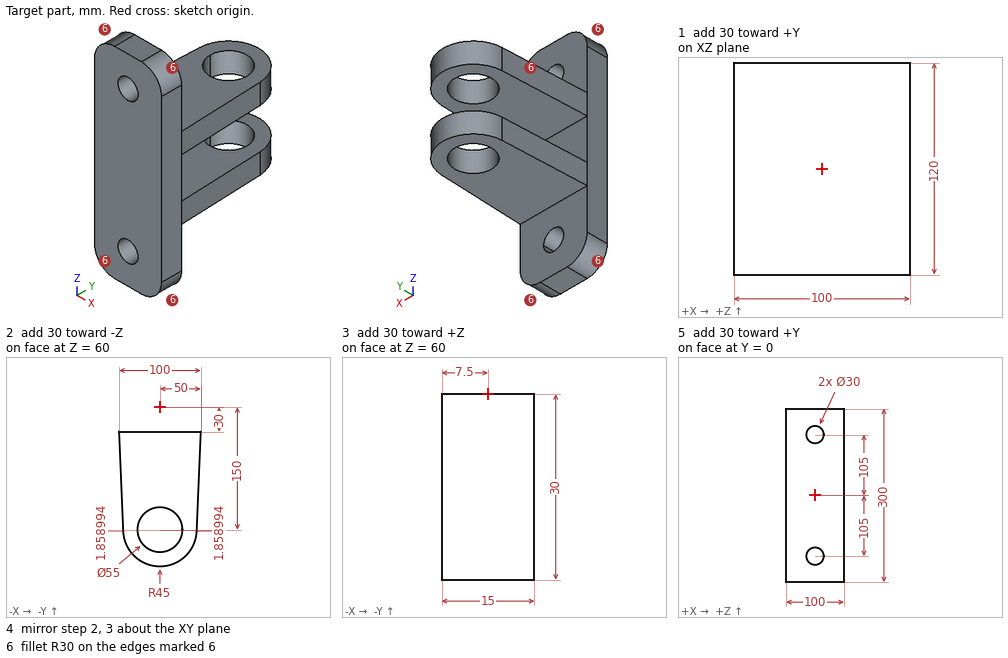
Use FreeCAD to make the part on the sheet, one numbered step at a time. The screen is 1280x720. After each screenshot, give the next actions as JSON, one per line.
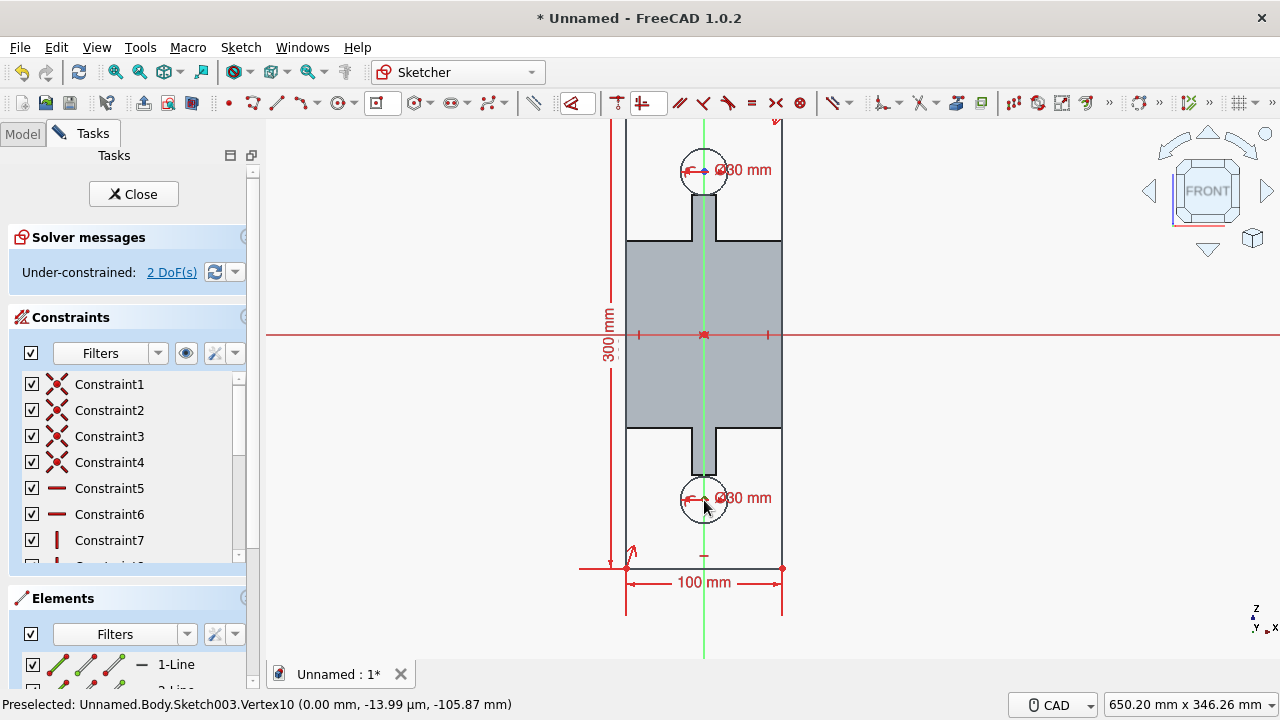
{"action": "left_click", "coordinate": [590, 104]}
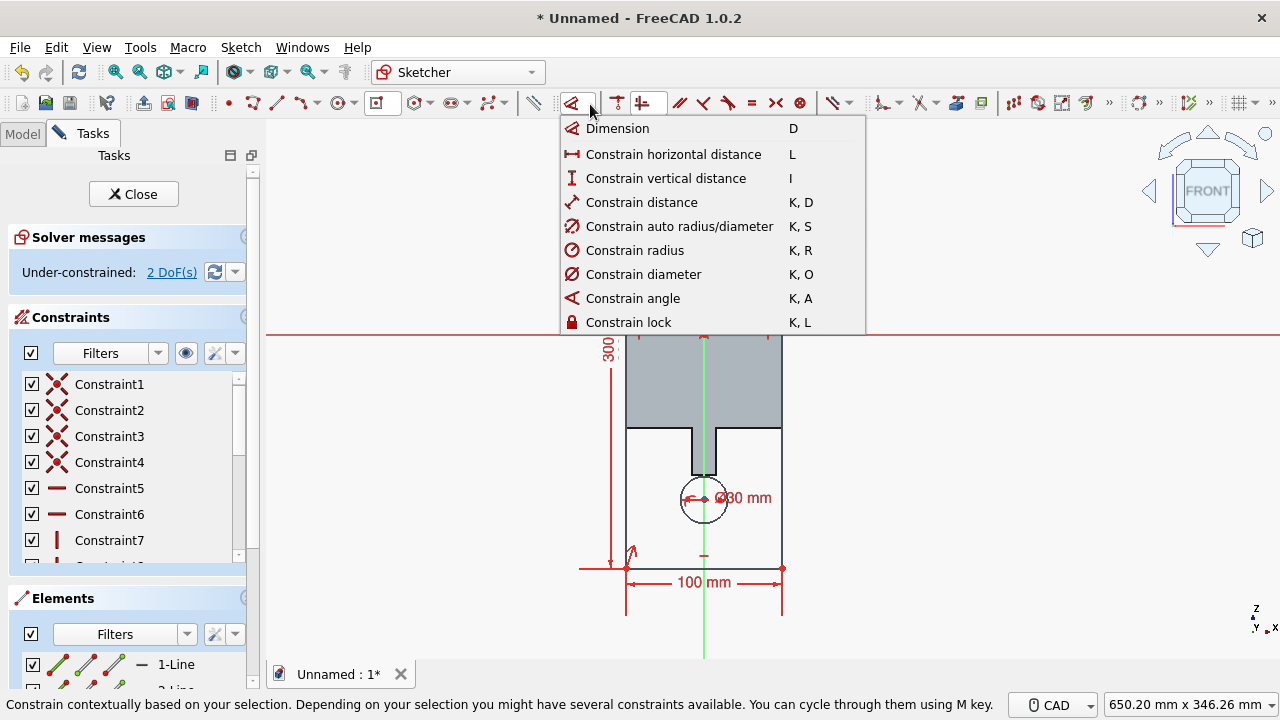
{"action": "left_click", "coordinate": [713, 178]}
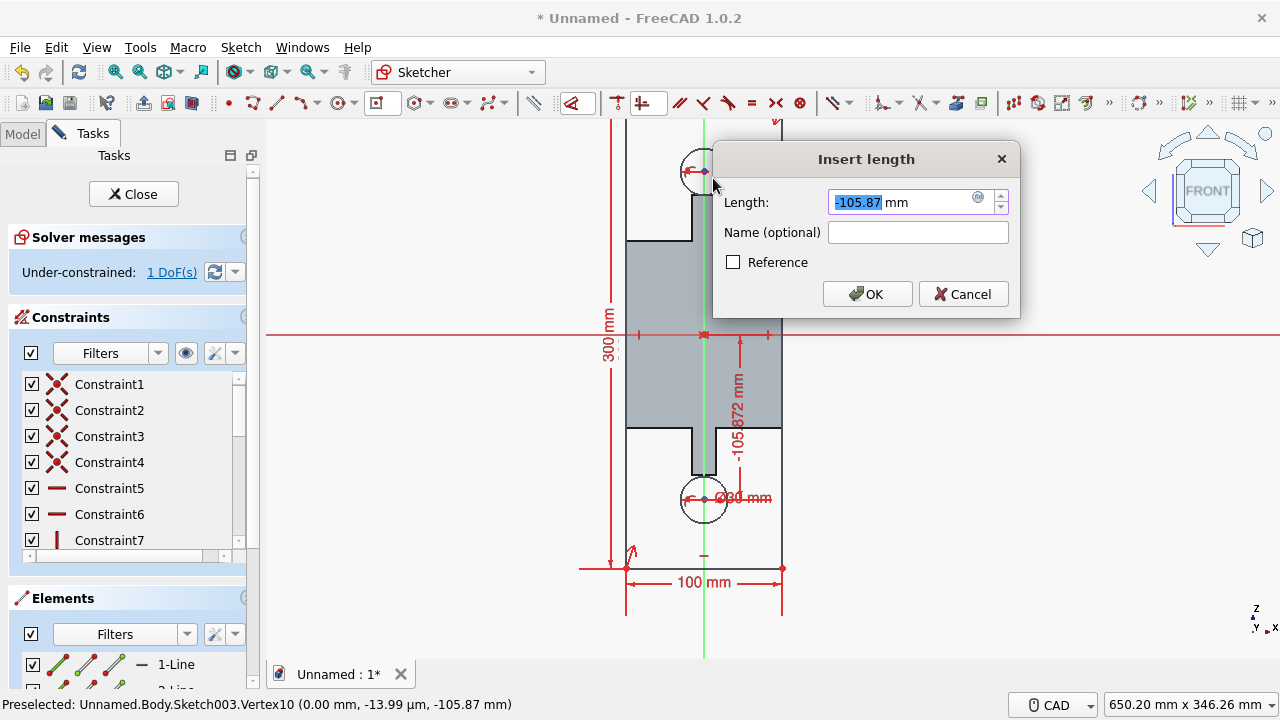
{"action": "type", "text": "-105"}
{"action": "key", "text": "Return"}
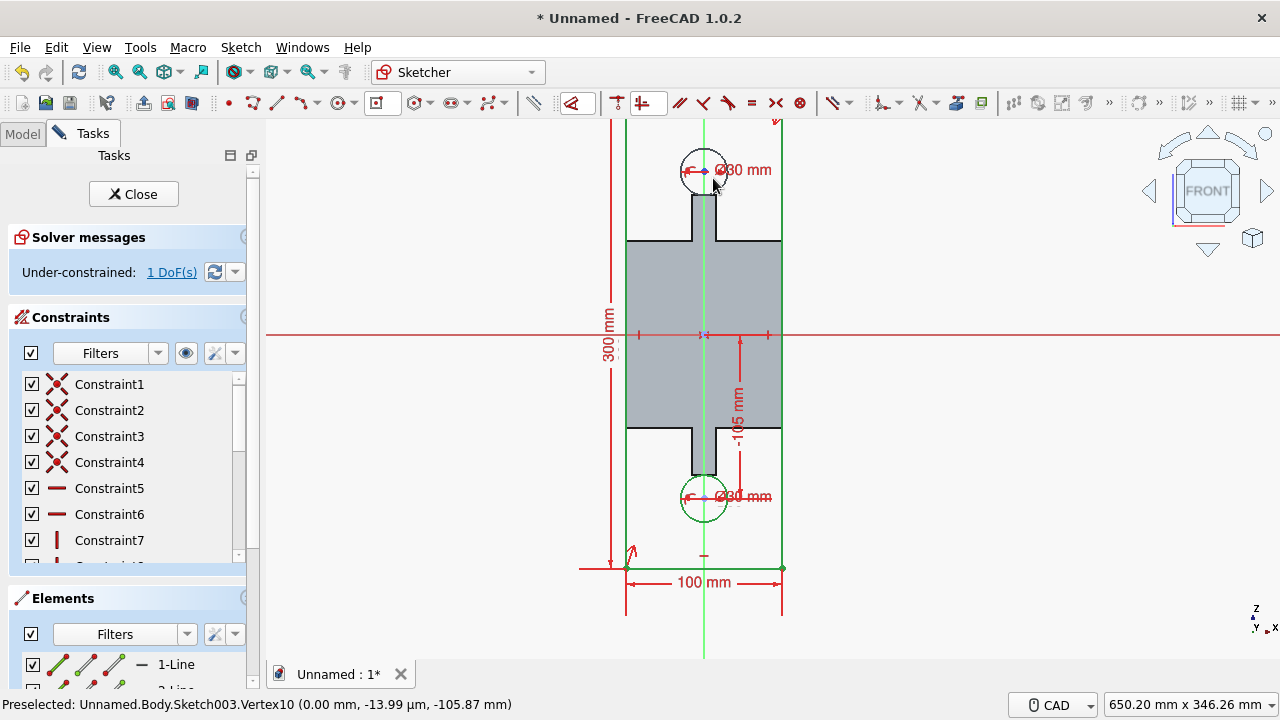
{"action": "left_click", "coordinate": [704, 172]}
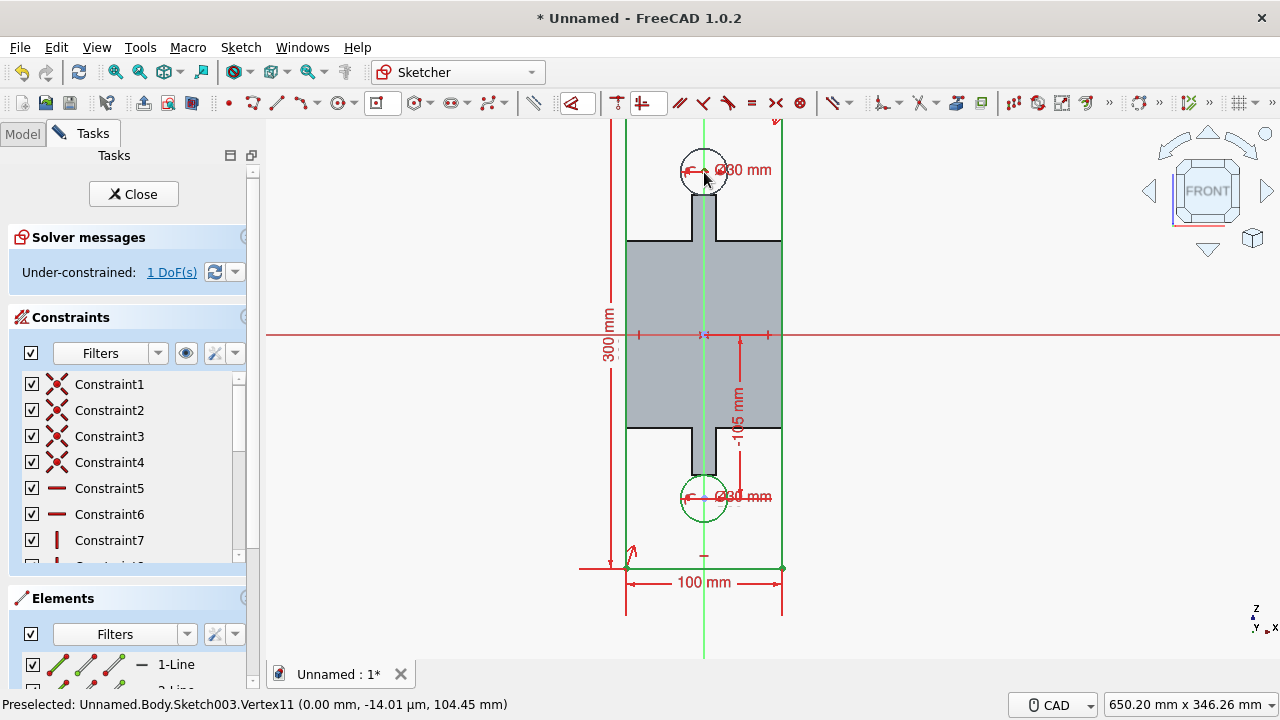
{"action": "key", "text": "i"}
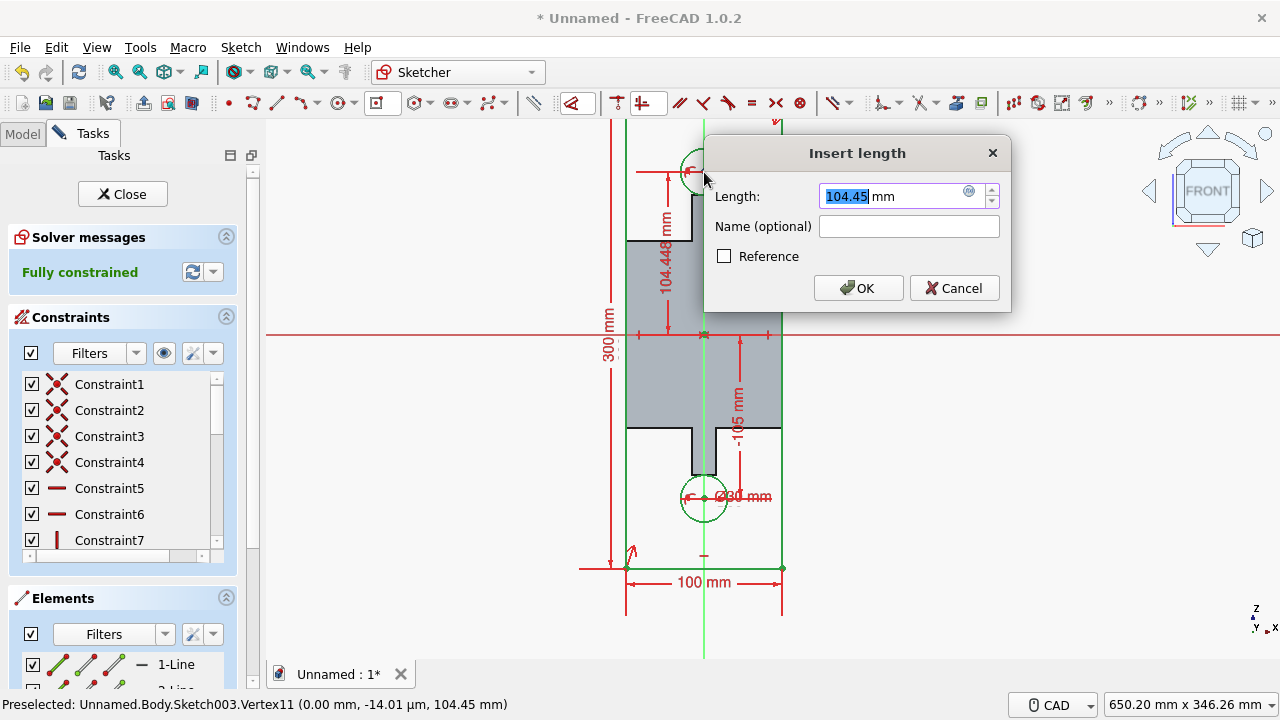
{"action": "type", "text": "105"}
{"action": "key", "text": "Return"}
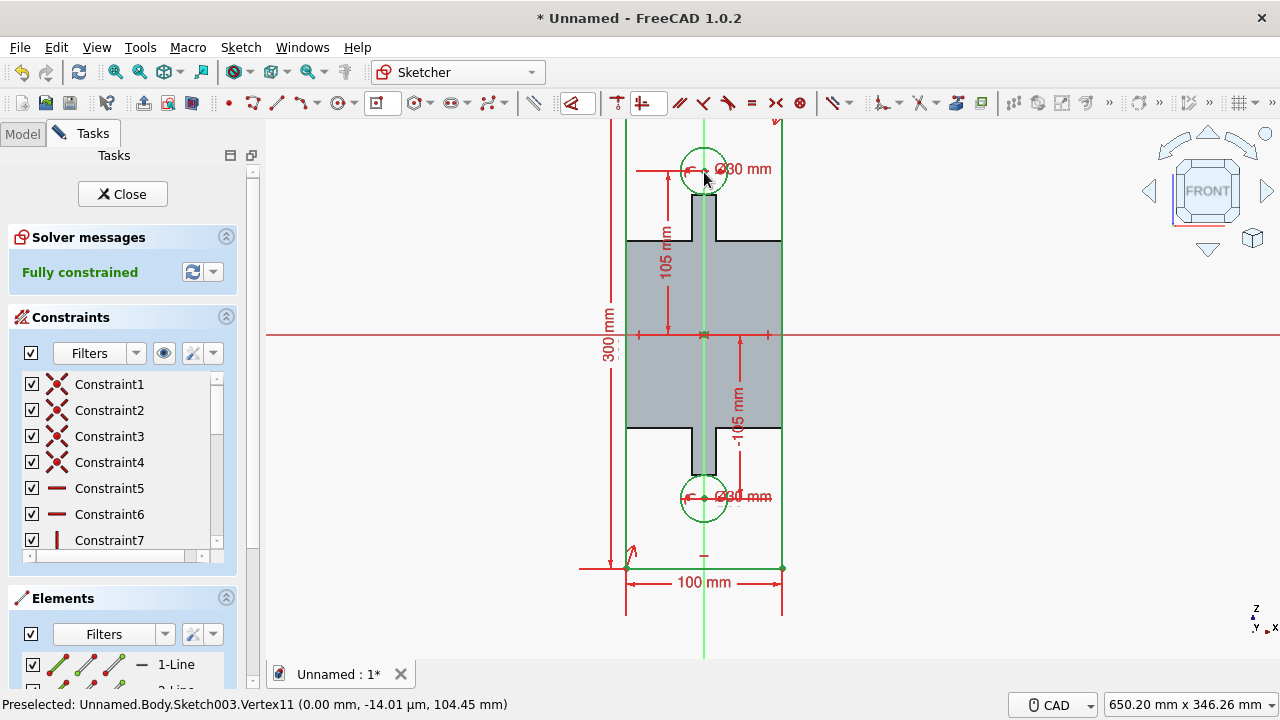
{"action": "left_click", "coordinate": [123, 194]}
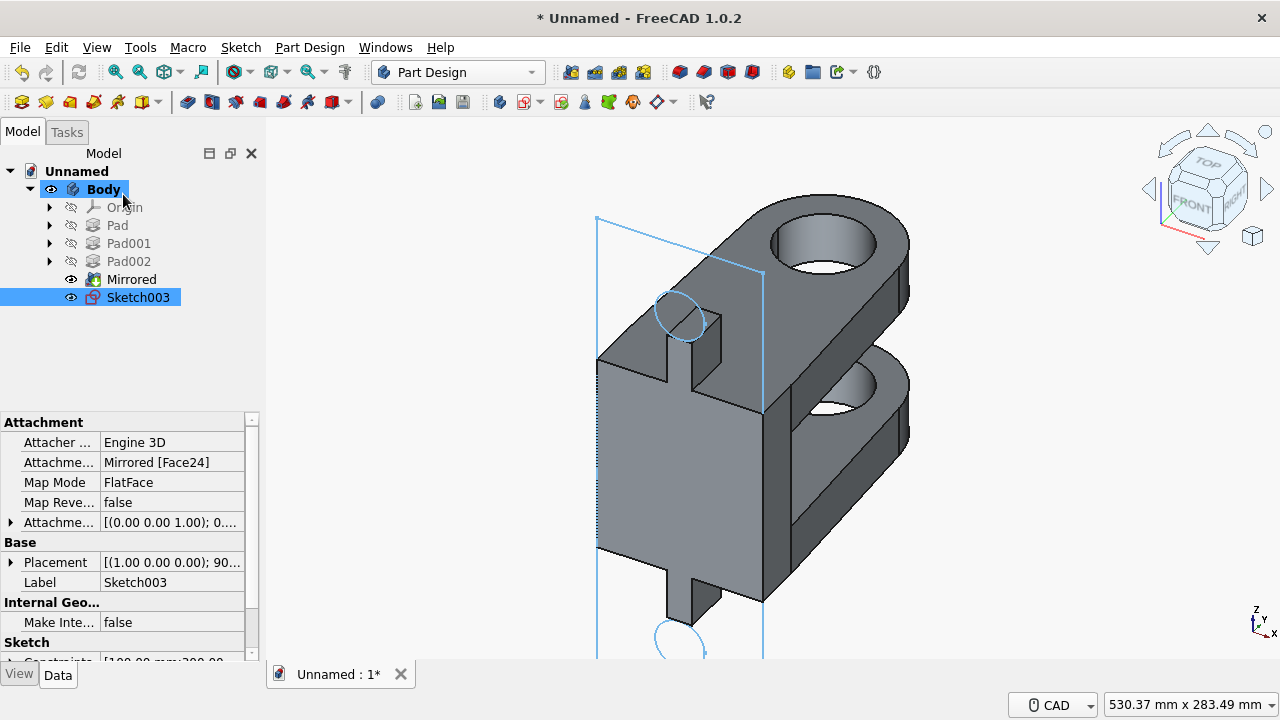
{"action": "left_click", "coordinate": [22, 102]}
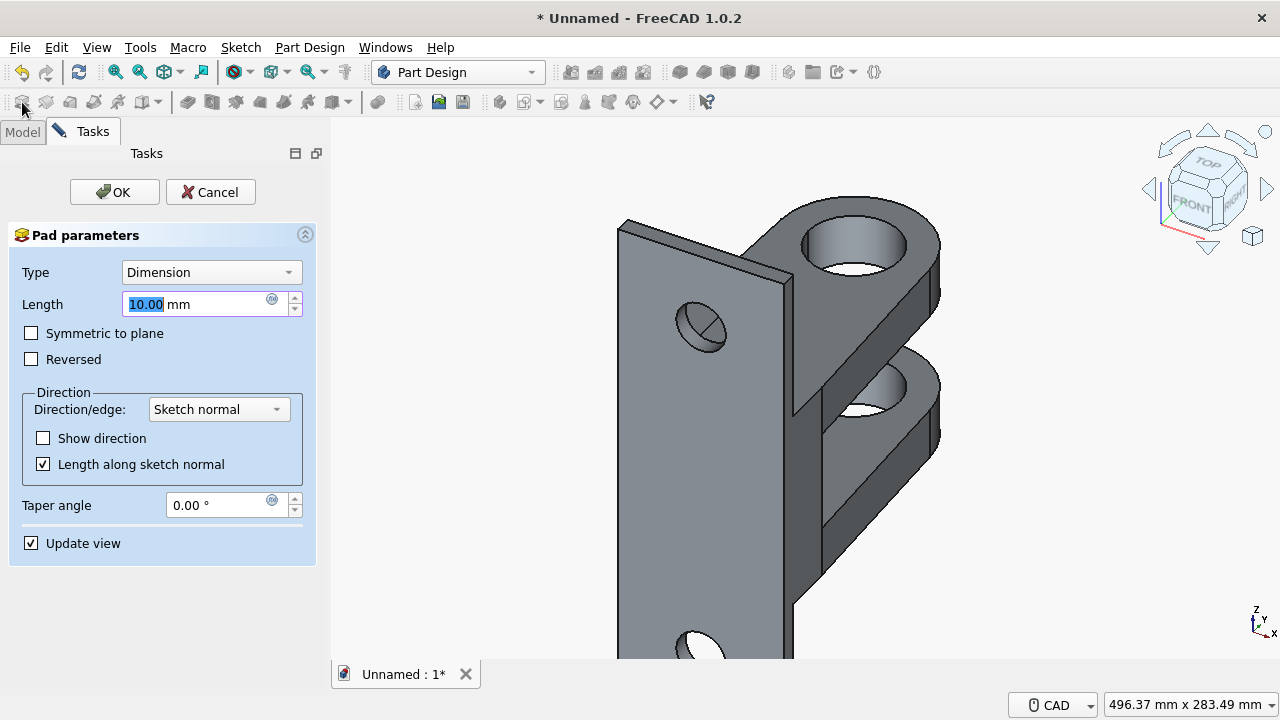
{"action": "type", "text": "30"}
{"action": "key", "text": "Tab"}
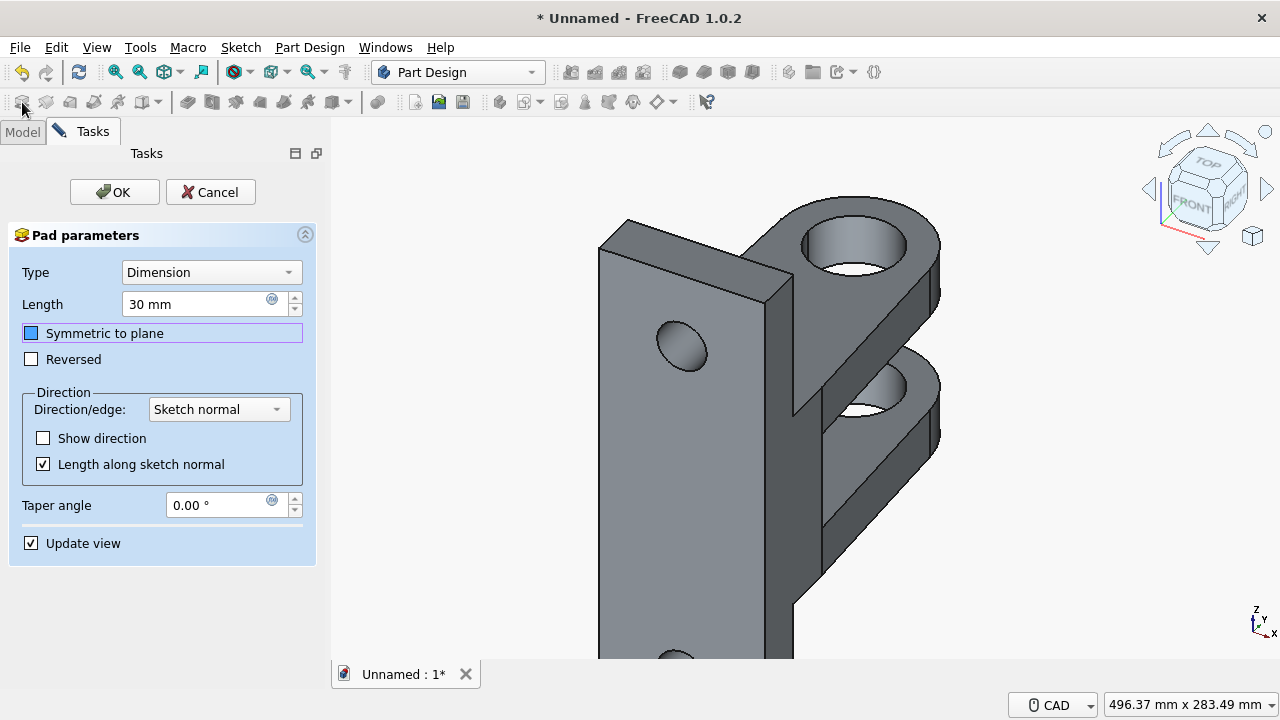
{"action": "left_click", "coordinate": [30, 359]}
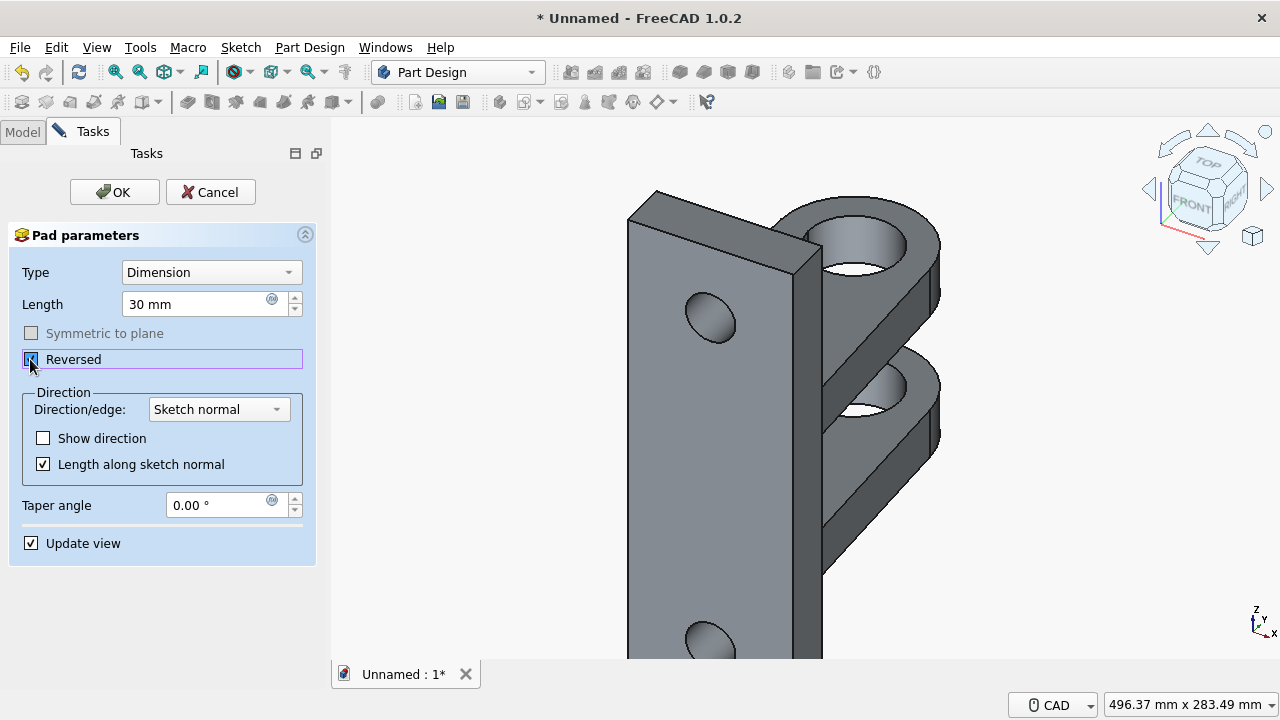
{"action": "left_click", "coordinate": [115, 192]}